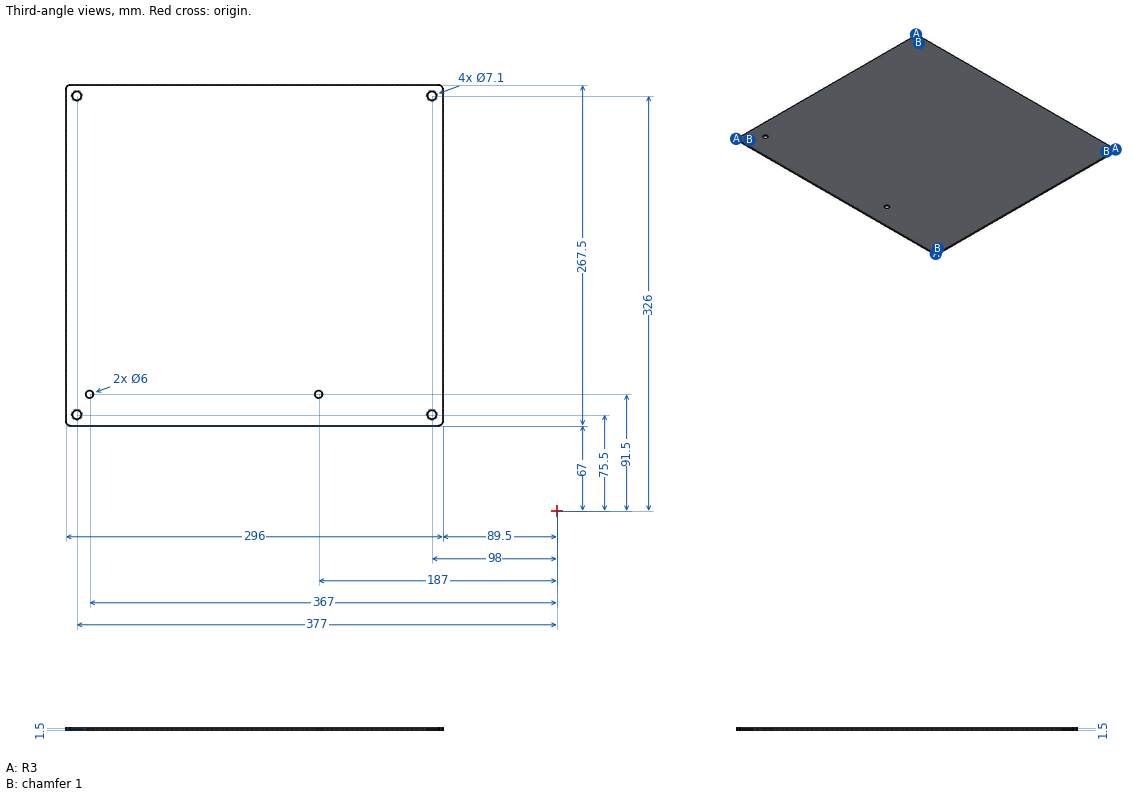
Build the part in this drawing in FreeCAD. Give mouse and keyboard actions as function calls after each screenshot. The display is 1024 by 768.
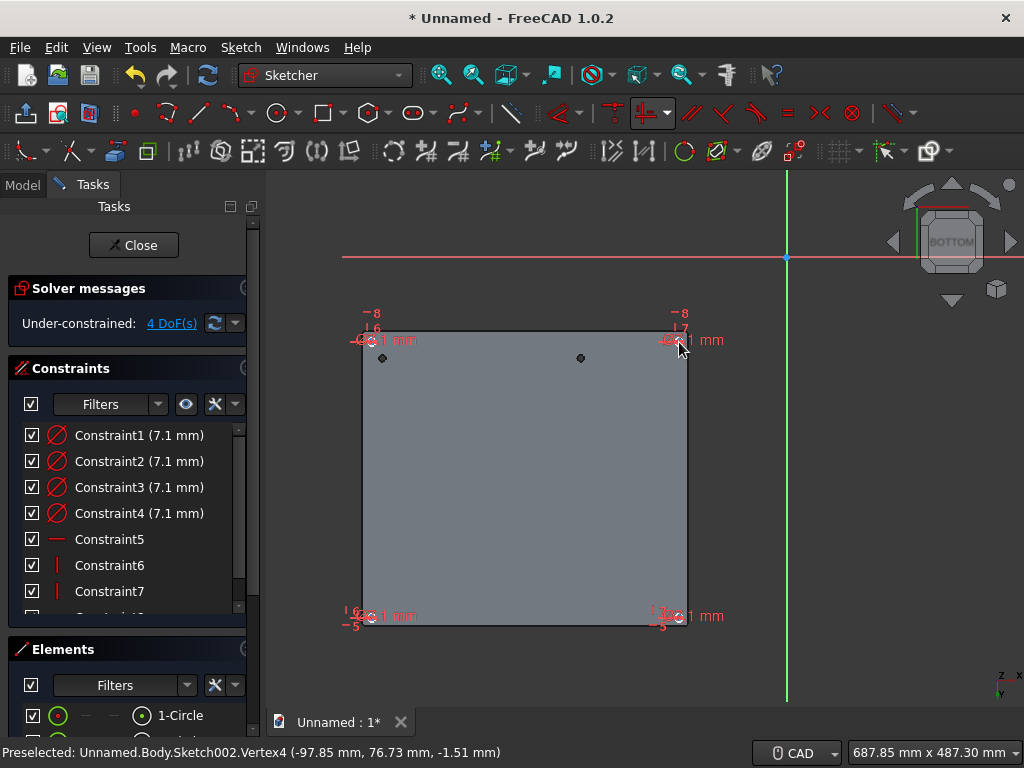
click(558, 114)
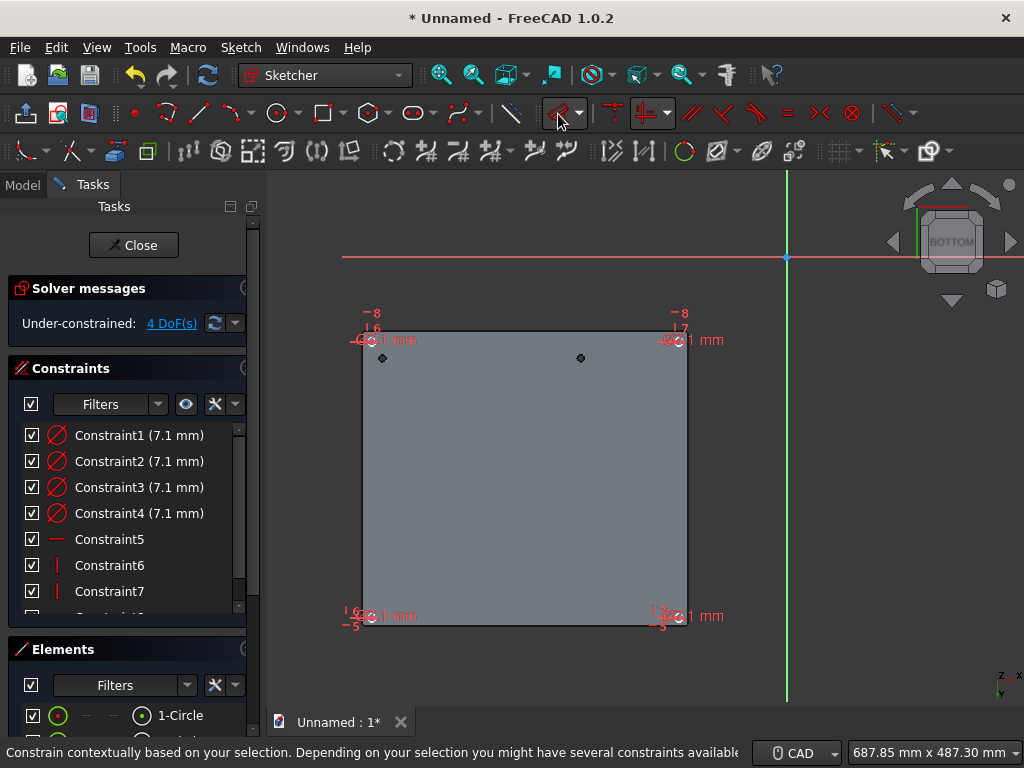
click(679, 618)
click(733, 223)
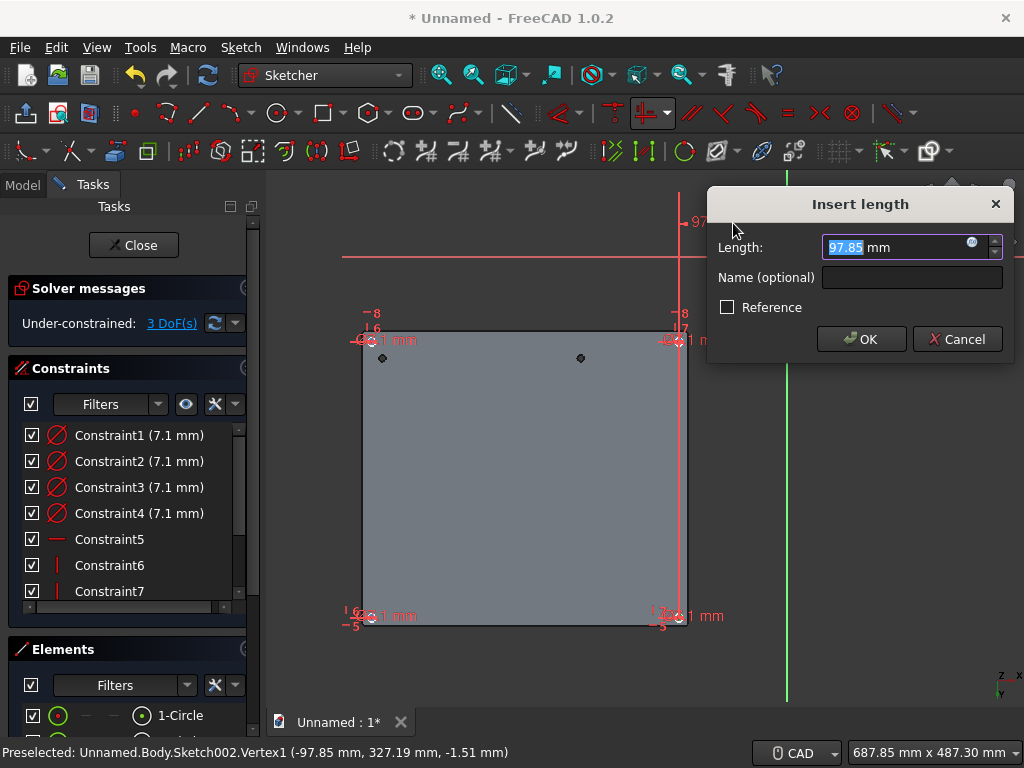
text(98)
key(Return)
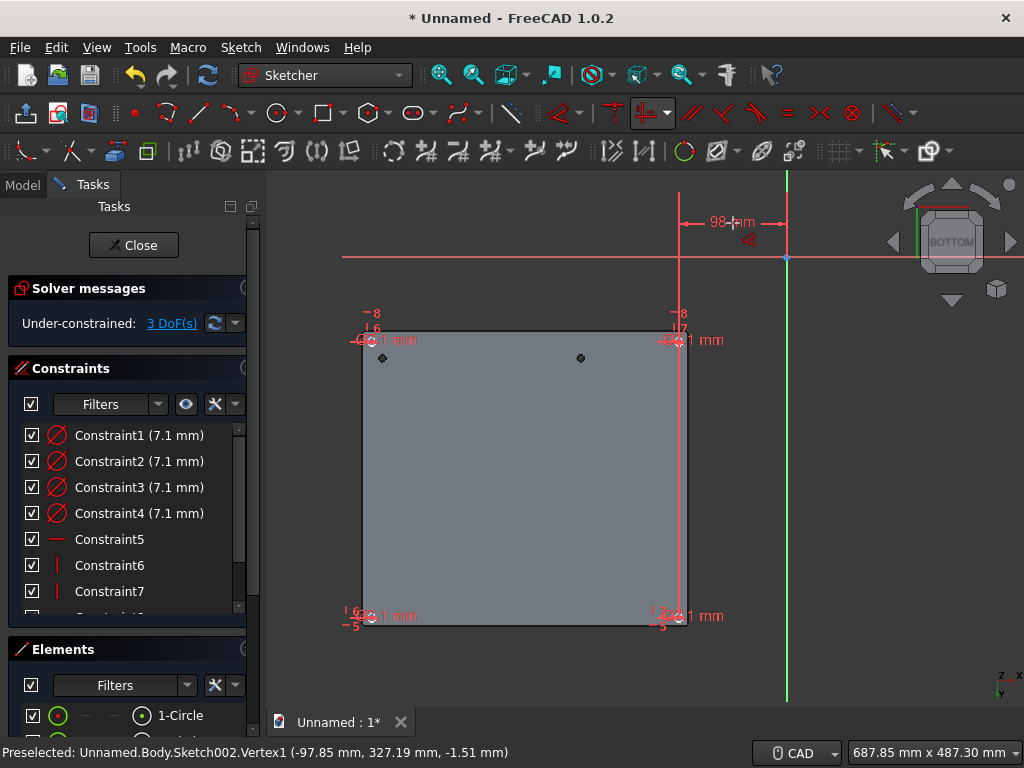
click(679, 618)
click(821, 438)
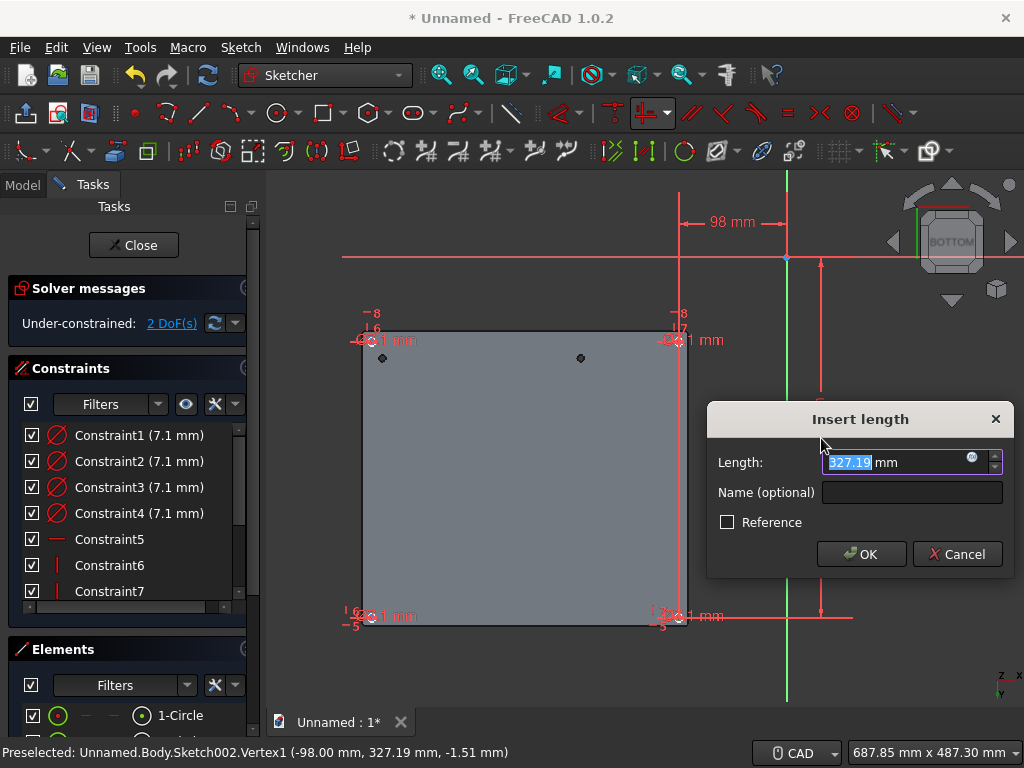
text(326)
key(Return)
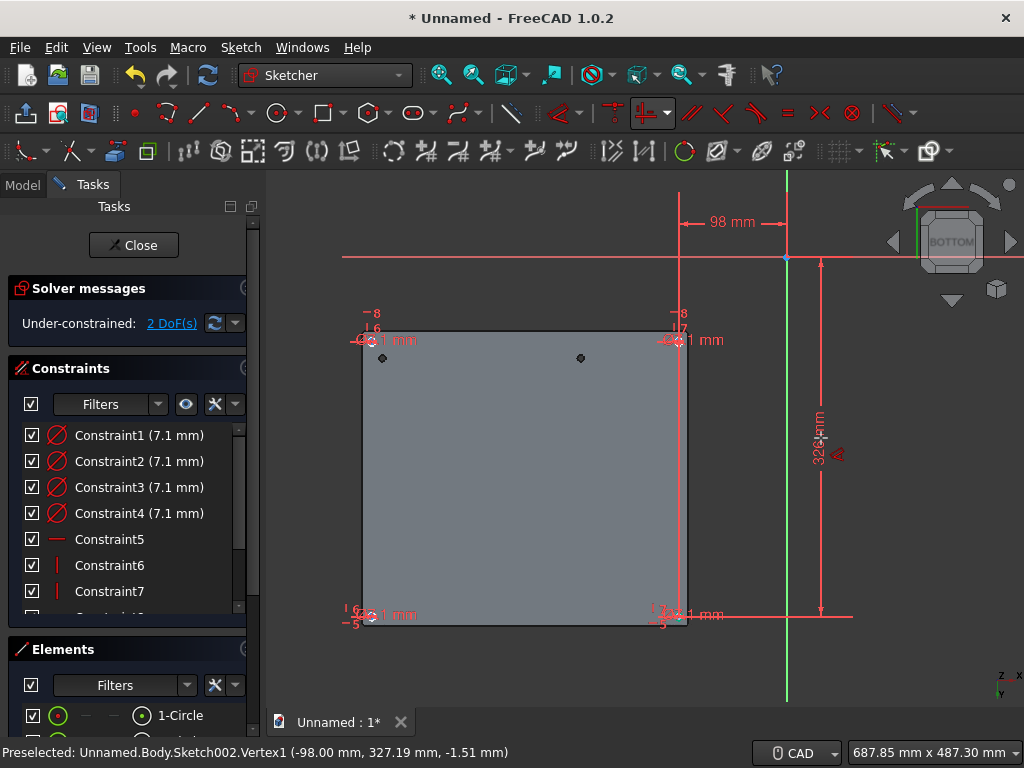
click(372, 617)
click(579, 223)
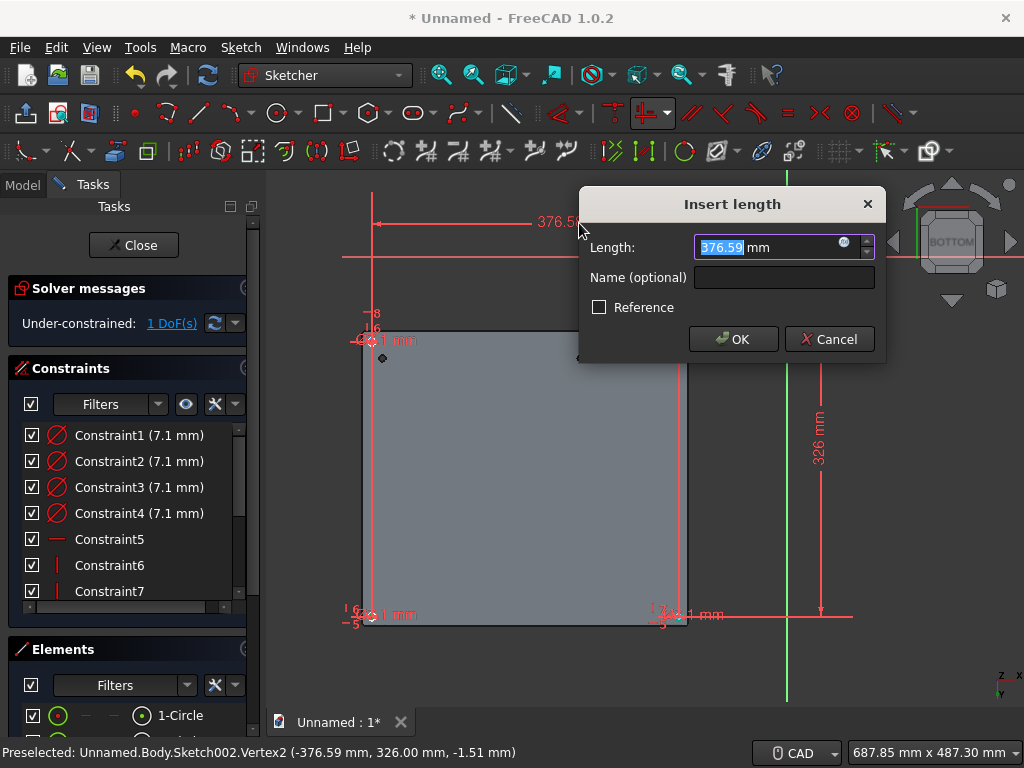
text(377)
key(Return)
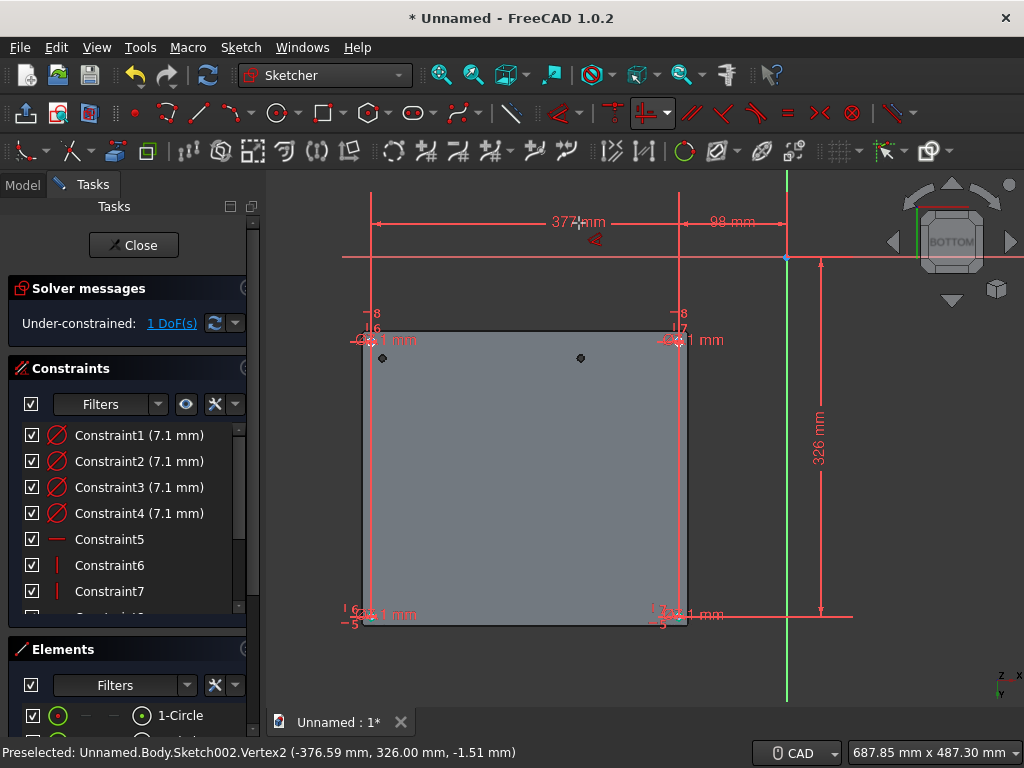
click(371, 342)
click(821, 300)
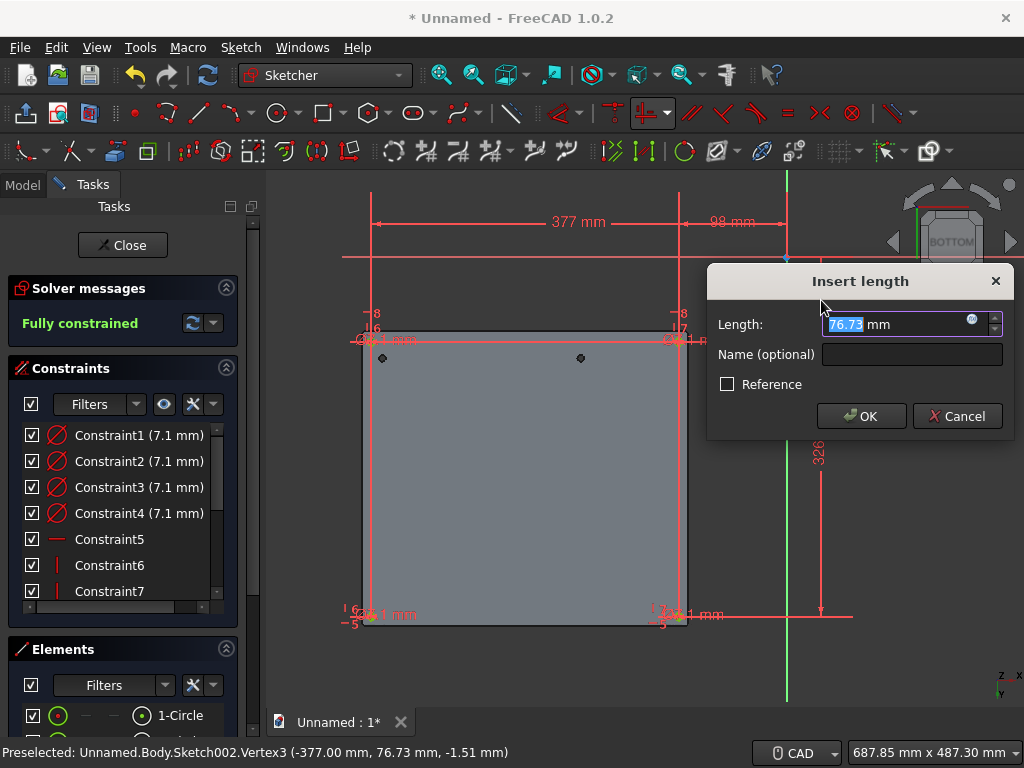
text(75.5)
key(Return)
key(Escape)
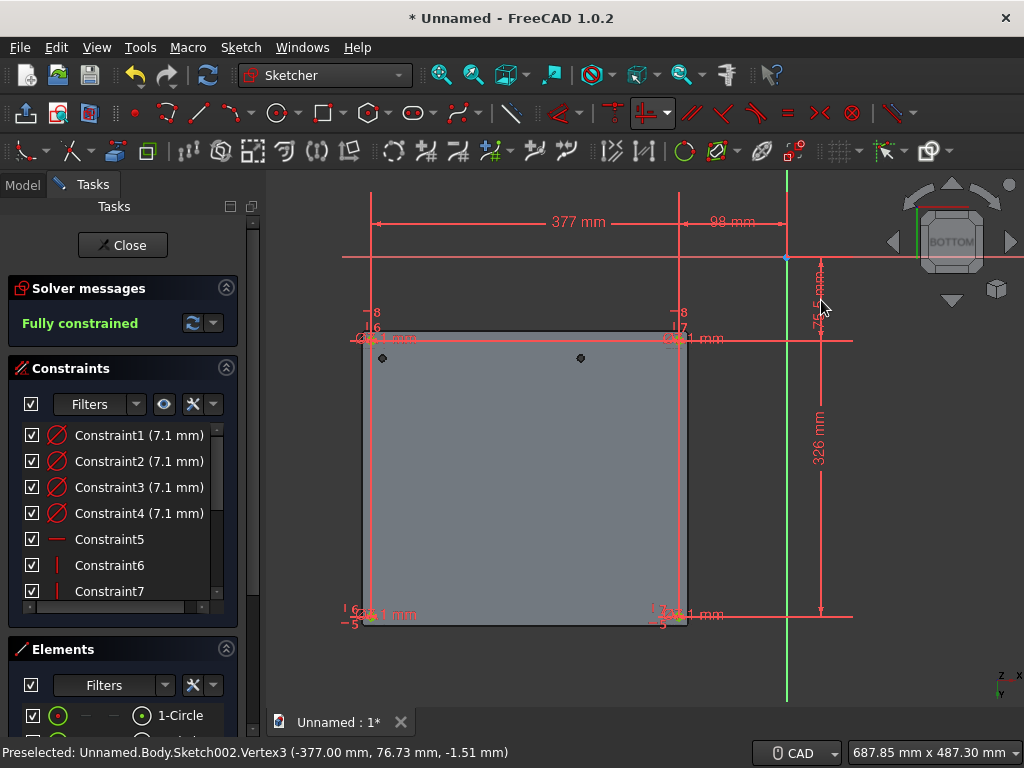
click(123, 245)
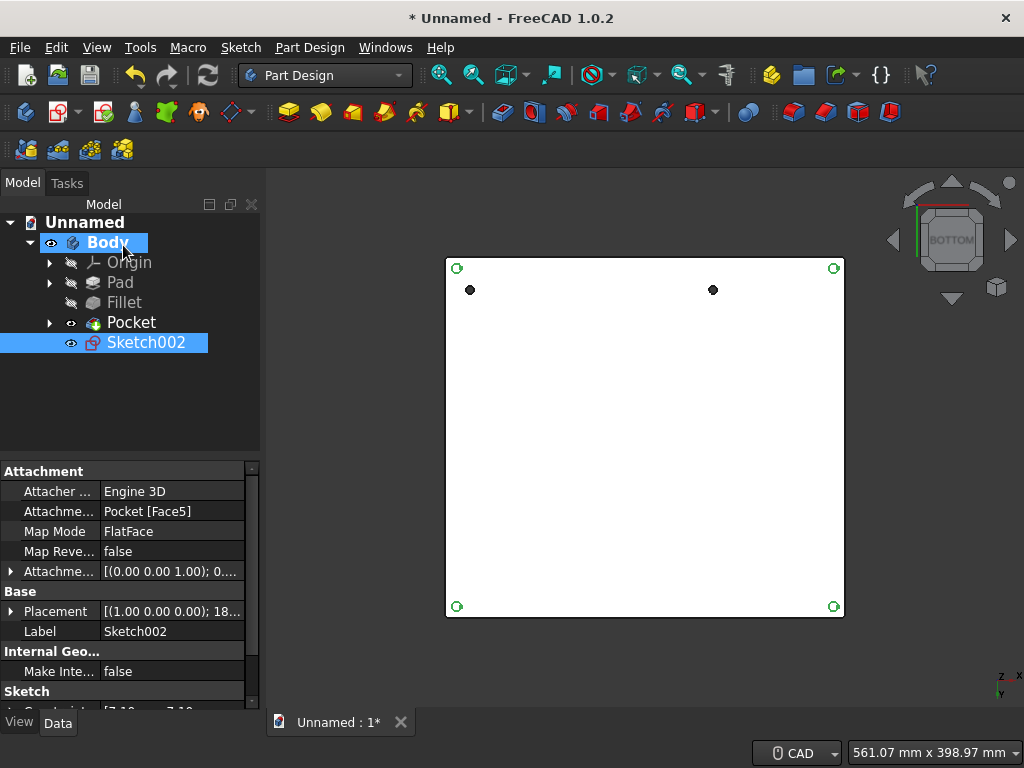
click(504, 112)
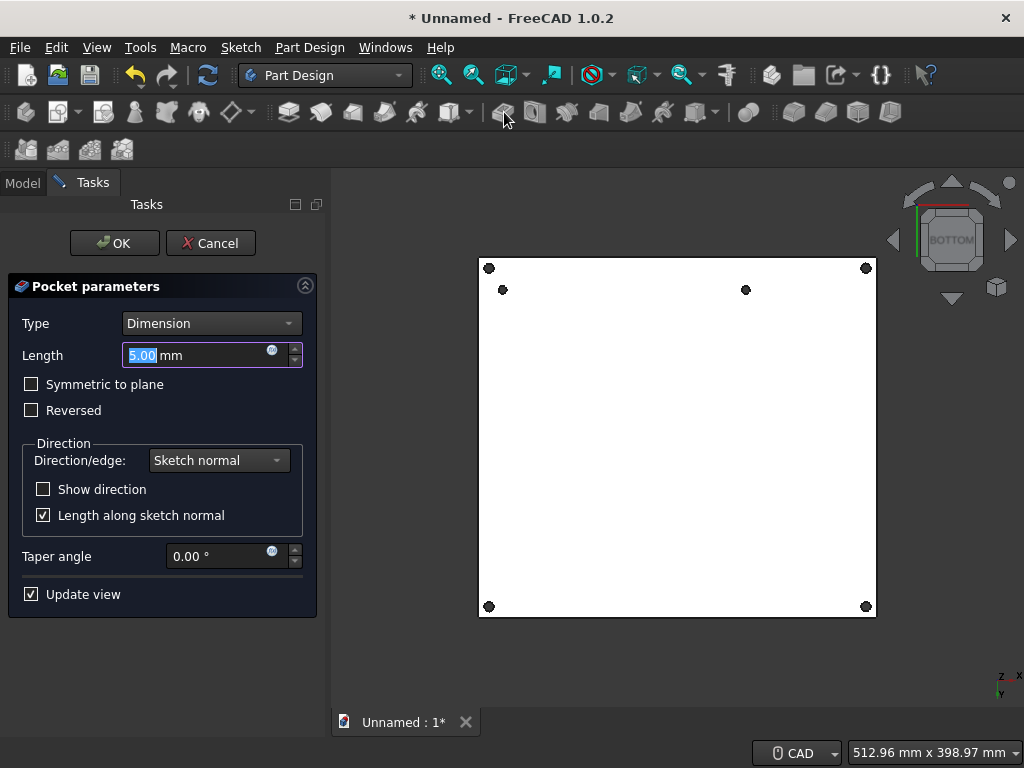
text(1.5)
key(Tab)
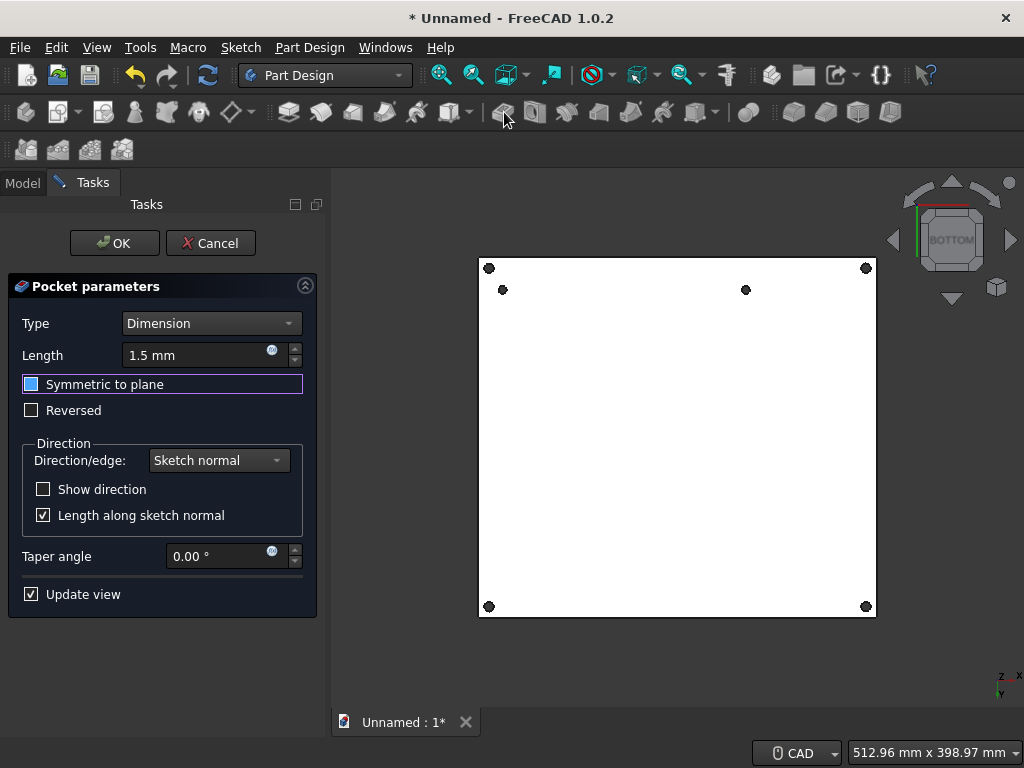
click(115, 243)